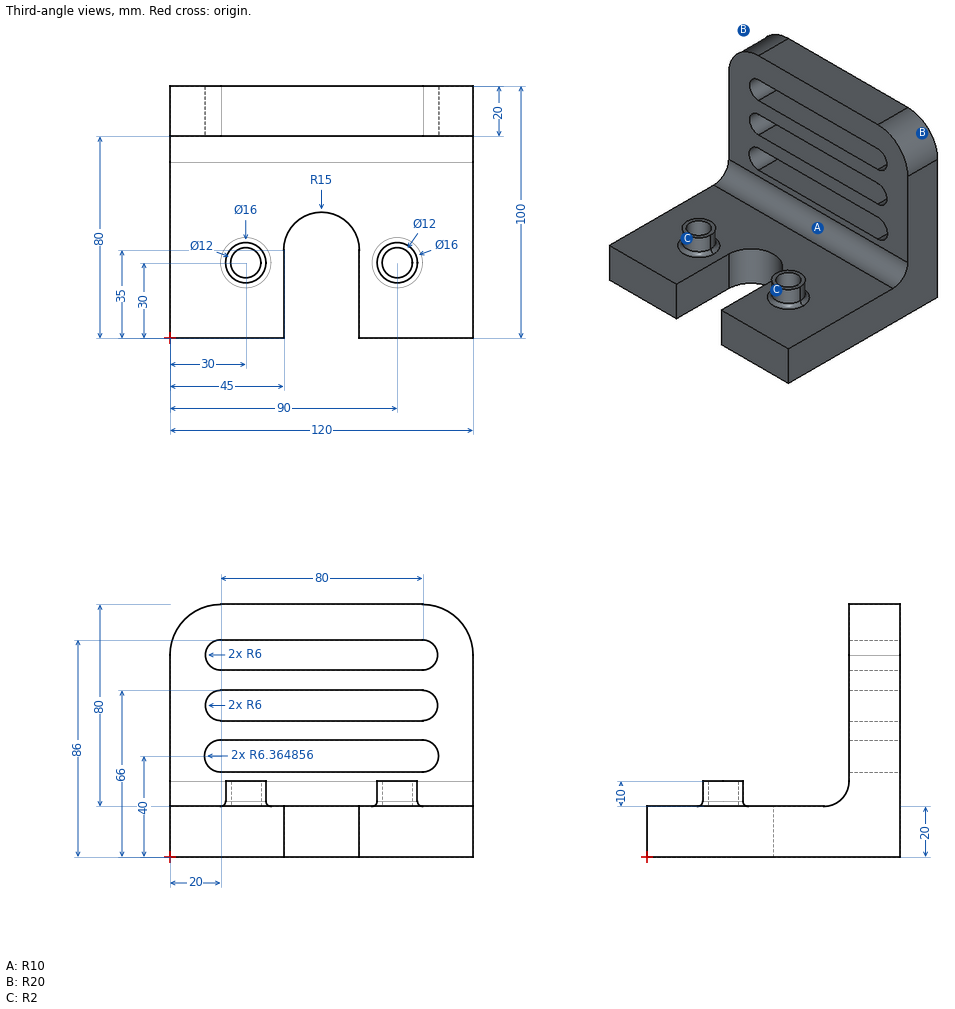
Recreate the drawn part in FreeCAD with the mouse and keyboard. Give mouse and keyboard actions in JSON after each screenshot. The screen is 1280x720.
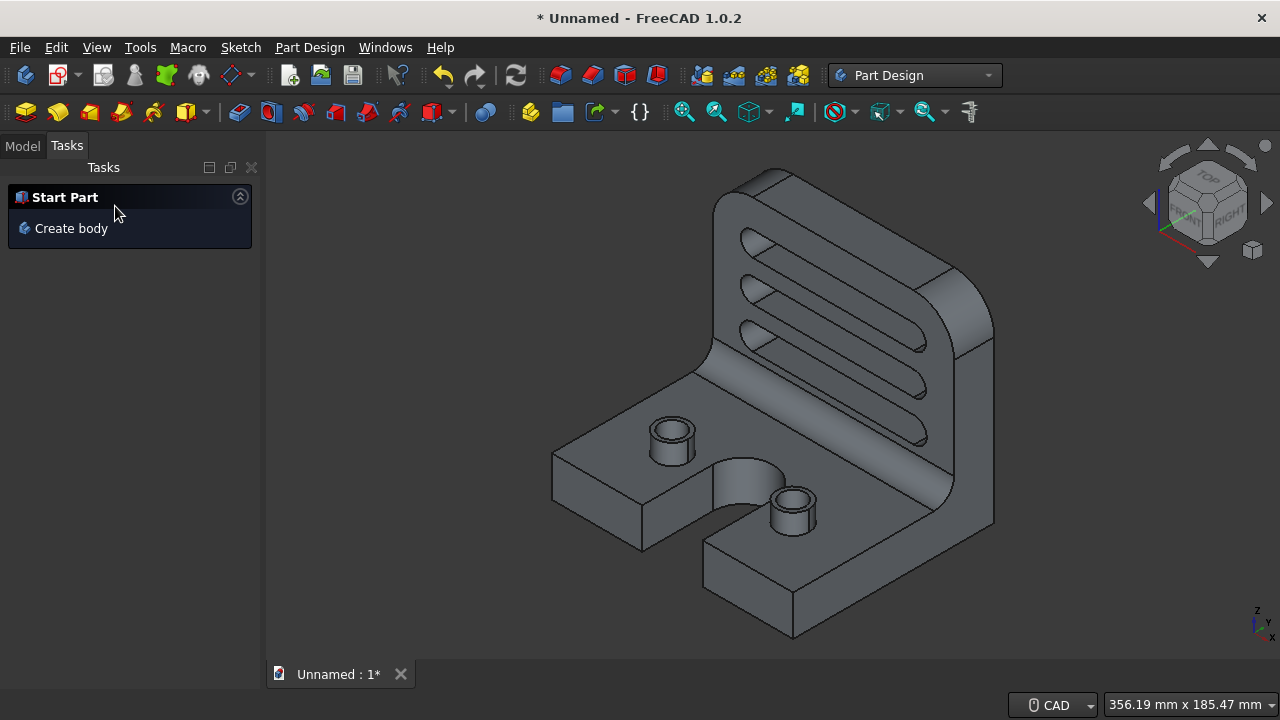
{"action": "left_click", "coordinate": [652, 458]}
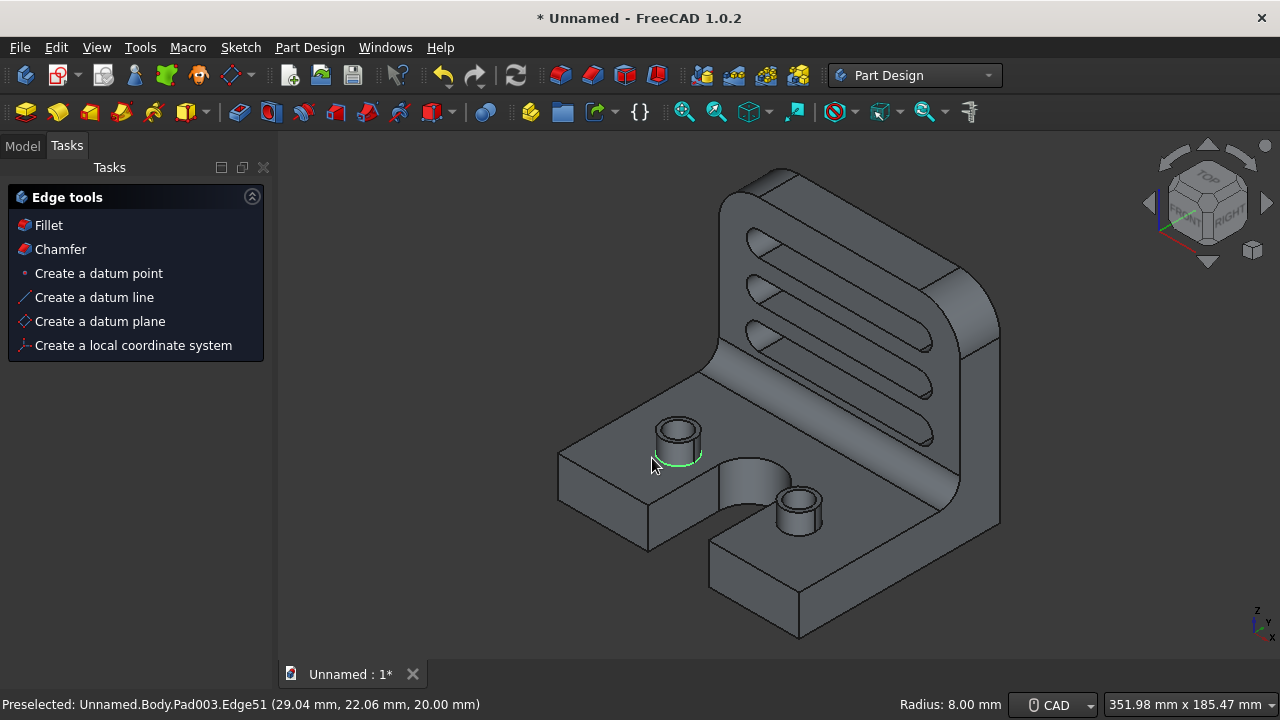
{"action": "left_click", "coordinate": [779, 528], "text": "ctrl"}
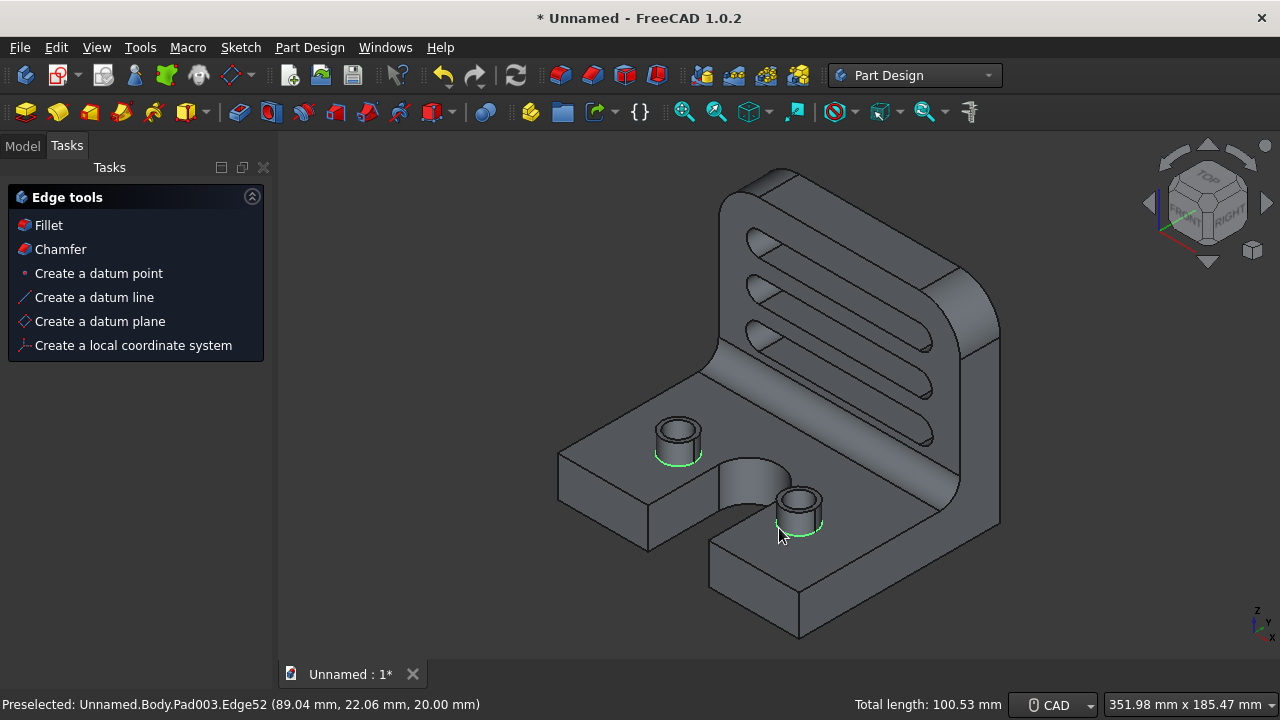
{"action": "left_click", "coordinate": [562, 76]}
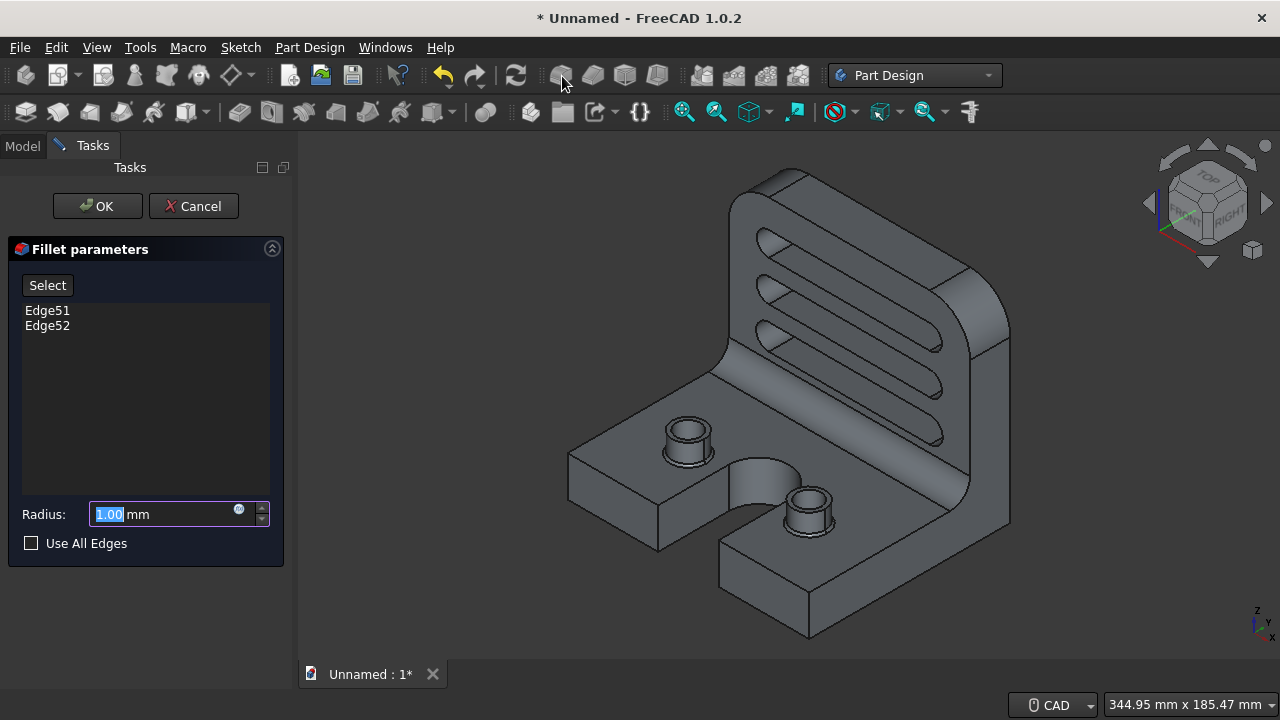
{"action": "type", "text": "2"}
{"action": "key", "text": "Tab"}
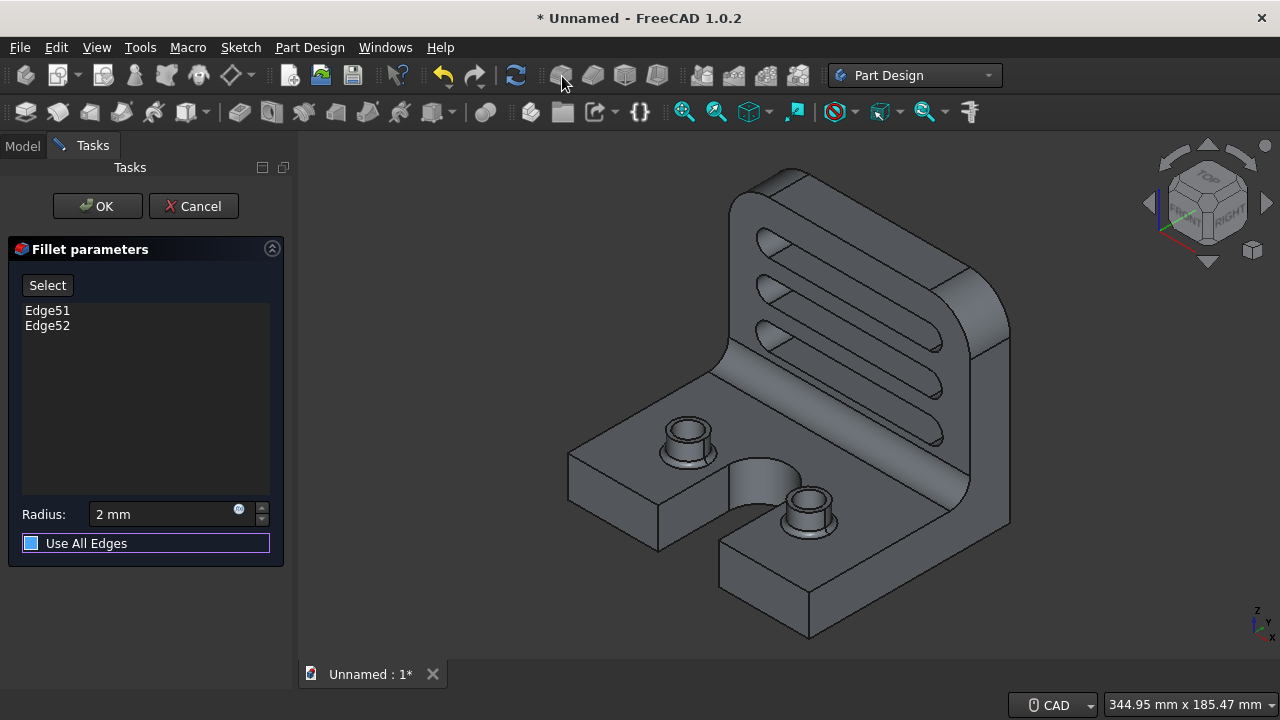
{"action": "left_click", "coordinate": [98, 206]}